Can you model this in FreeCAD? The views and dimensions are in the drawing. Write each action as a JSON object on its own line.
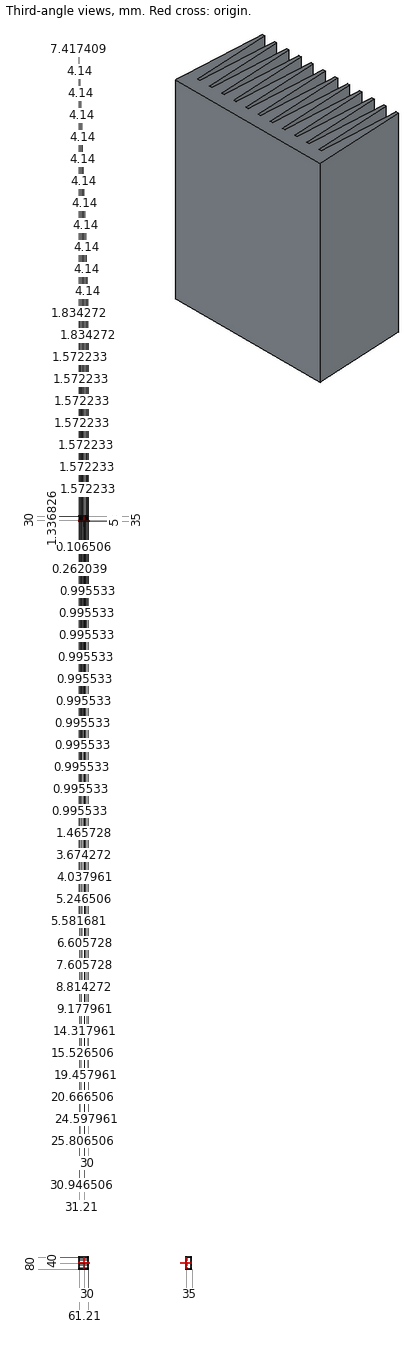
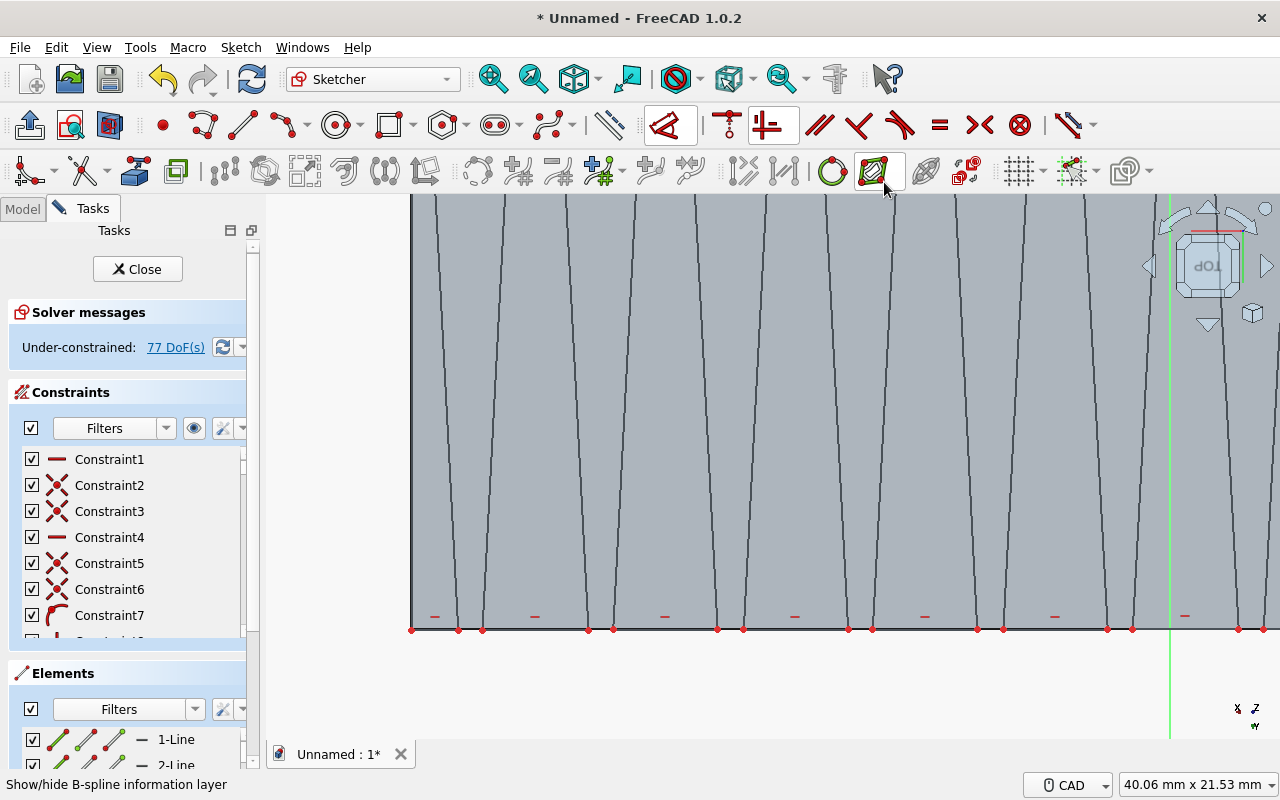
{"action": "scroll", "coordinate": [424, 630], "scroll_direction": "down", "scroll_amount": 5}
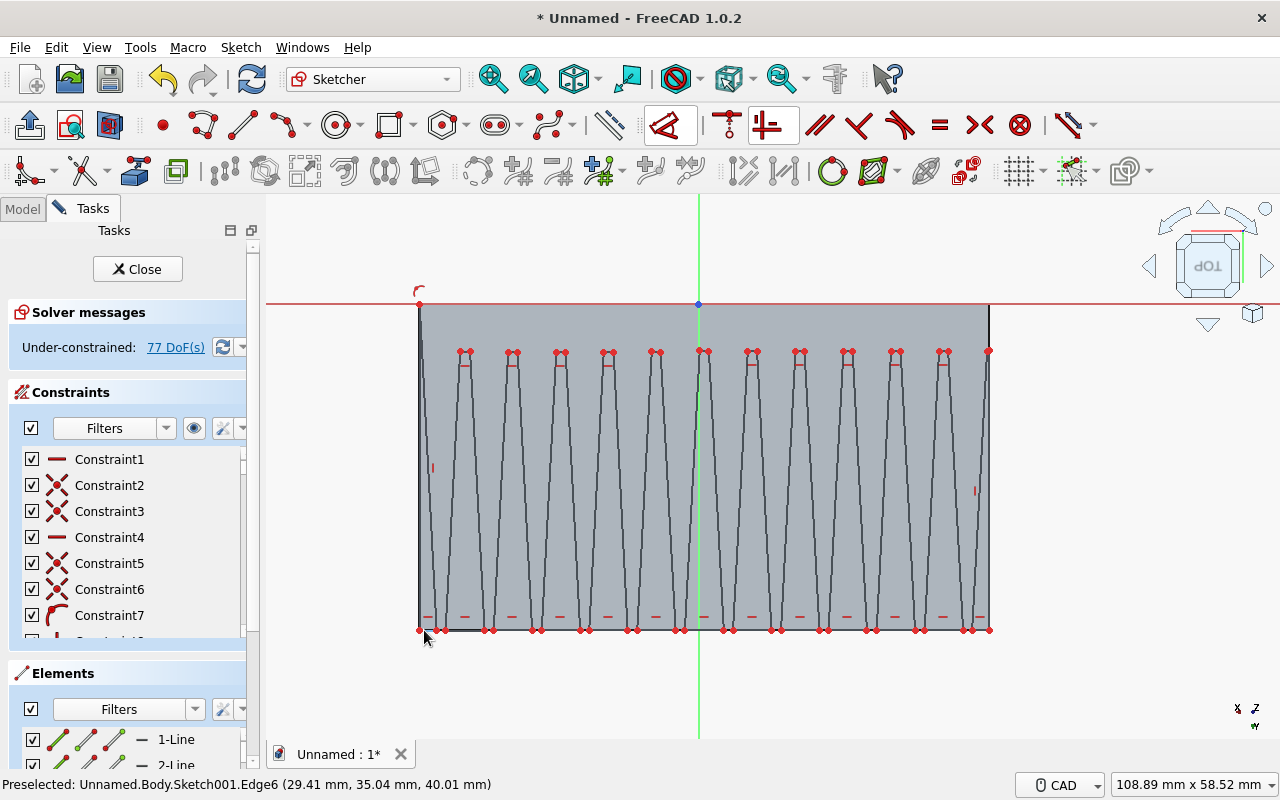
{"action": "scroll", "coordinate": [657, 352], "scroll_direction": "up", "scroll_amount": 7}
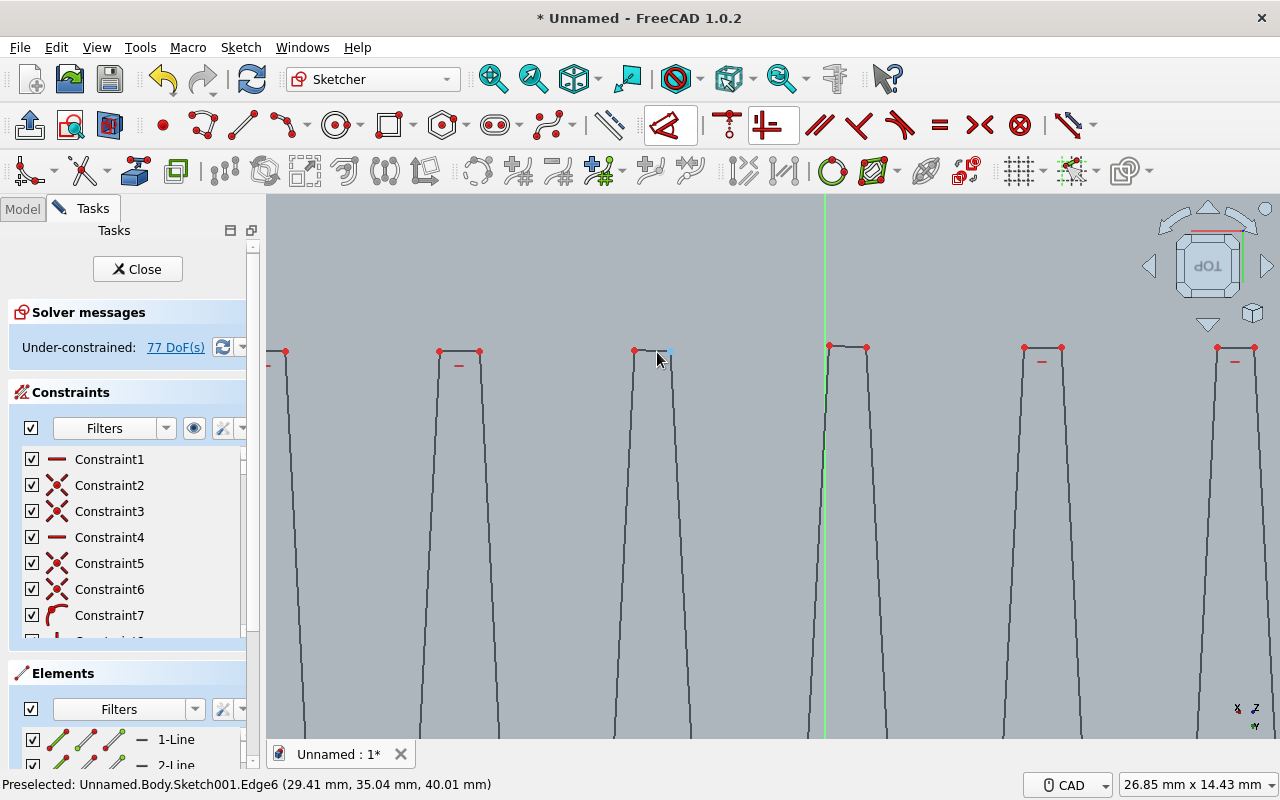
{"action": "left_click", "coordinate": [656, 351]}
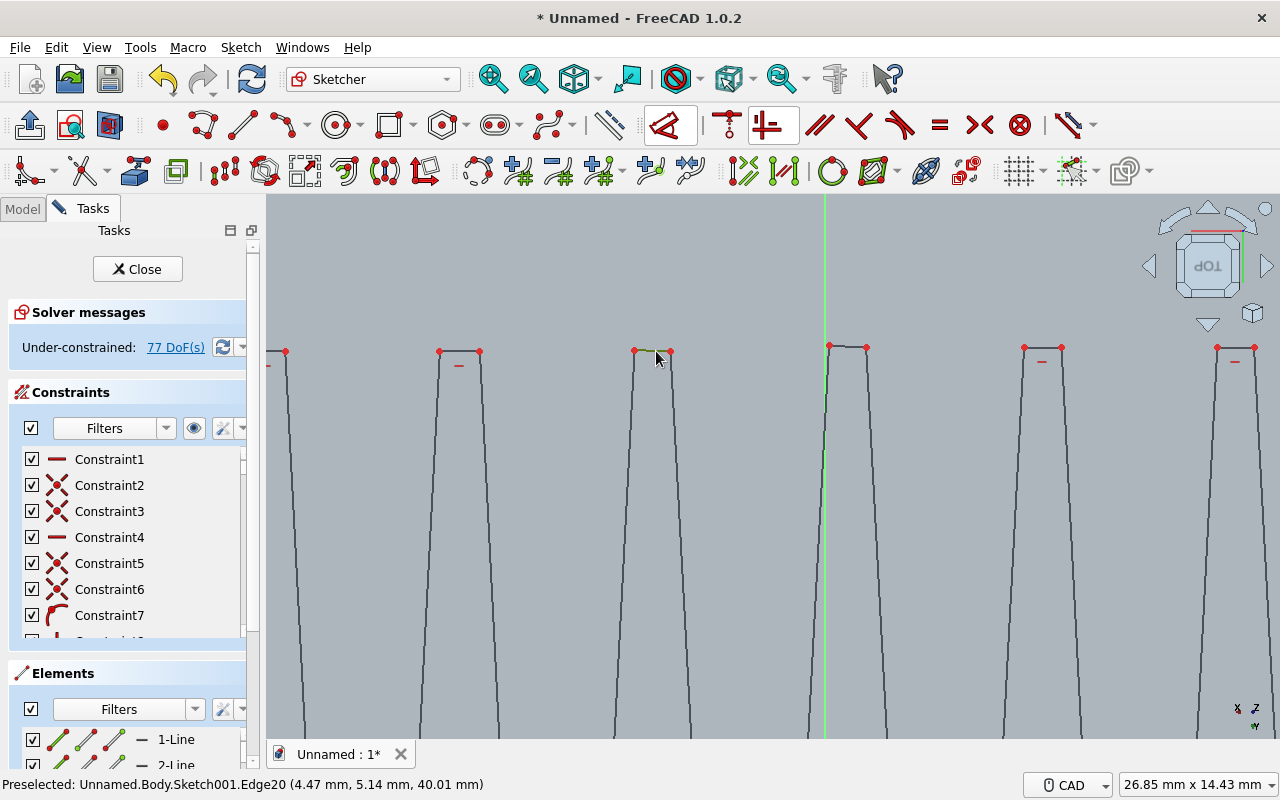
{"action": "key", "text": "h"}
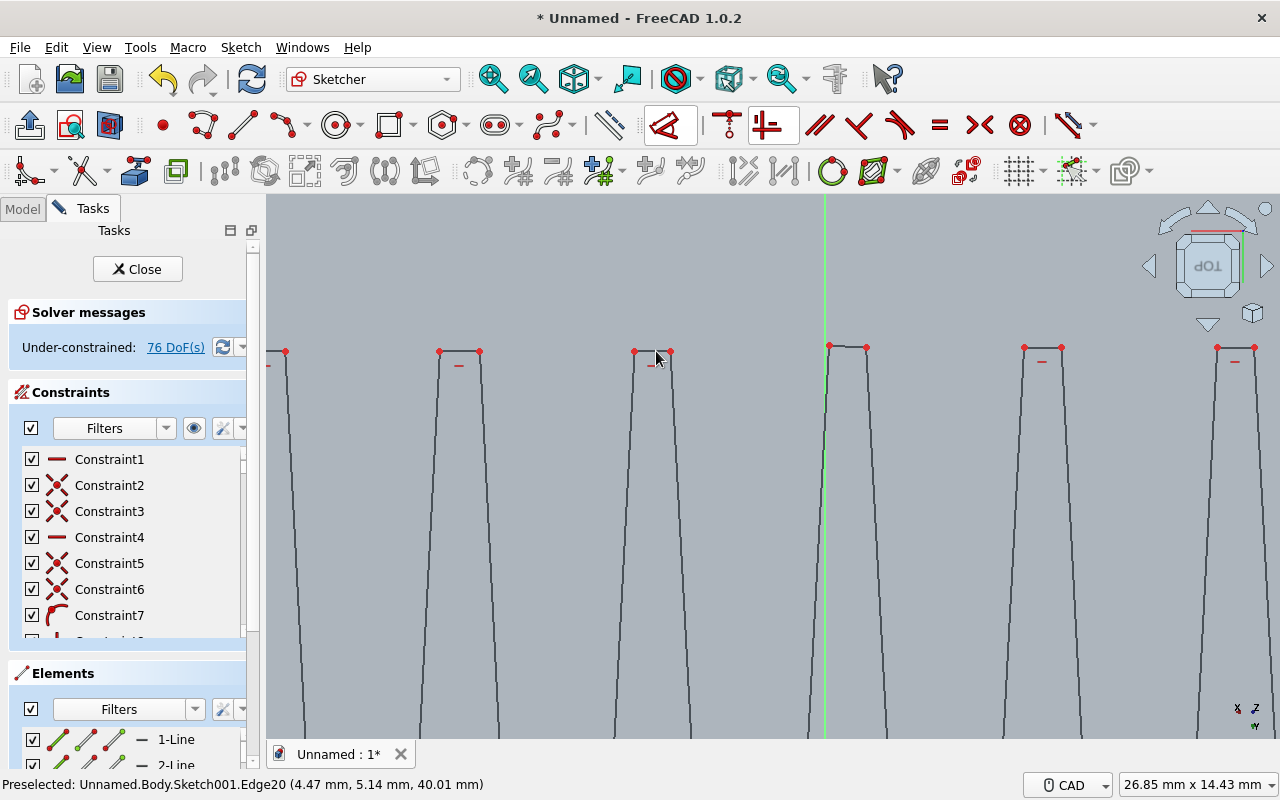
{"action": "scroll", "coordinate": [855, 347], "scroll_direction": "up", "scroll_amount": 2}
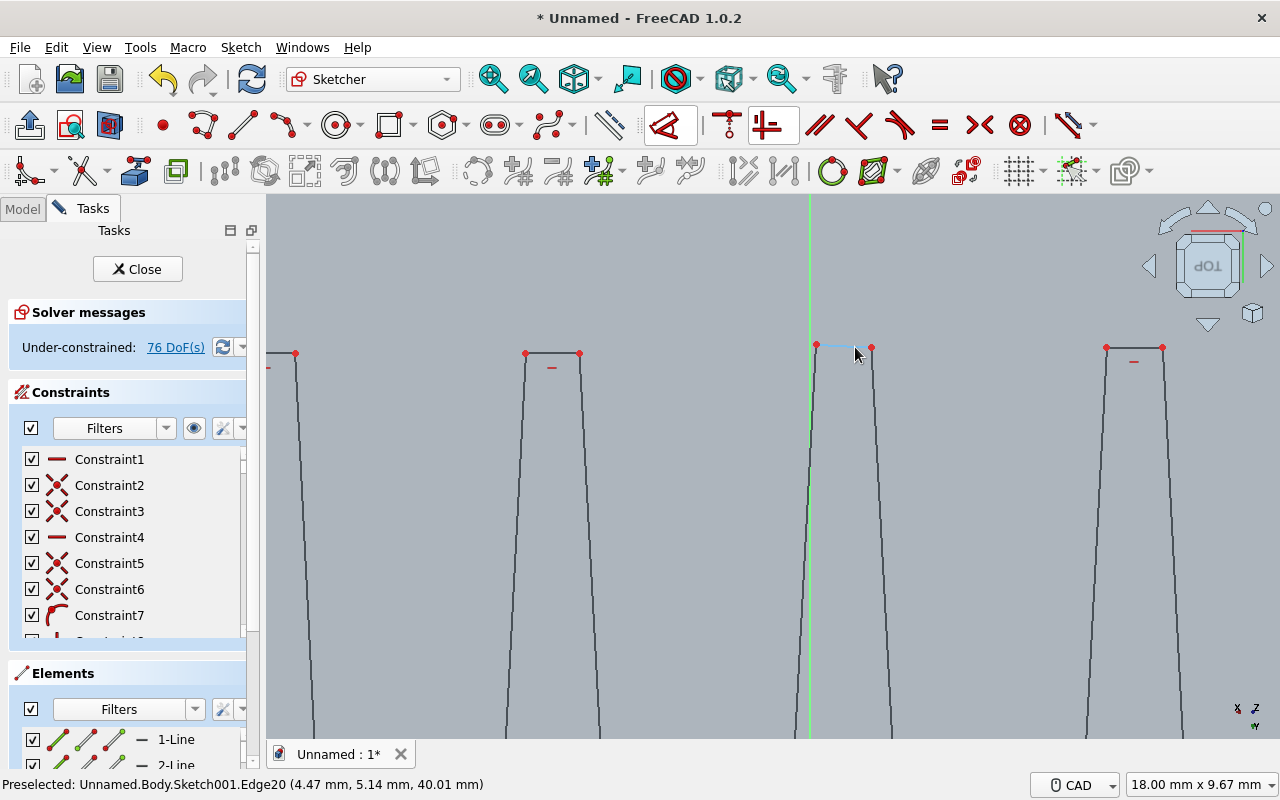
{"action": "left_click", "coordinate": [855, 347]}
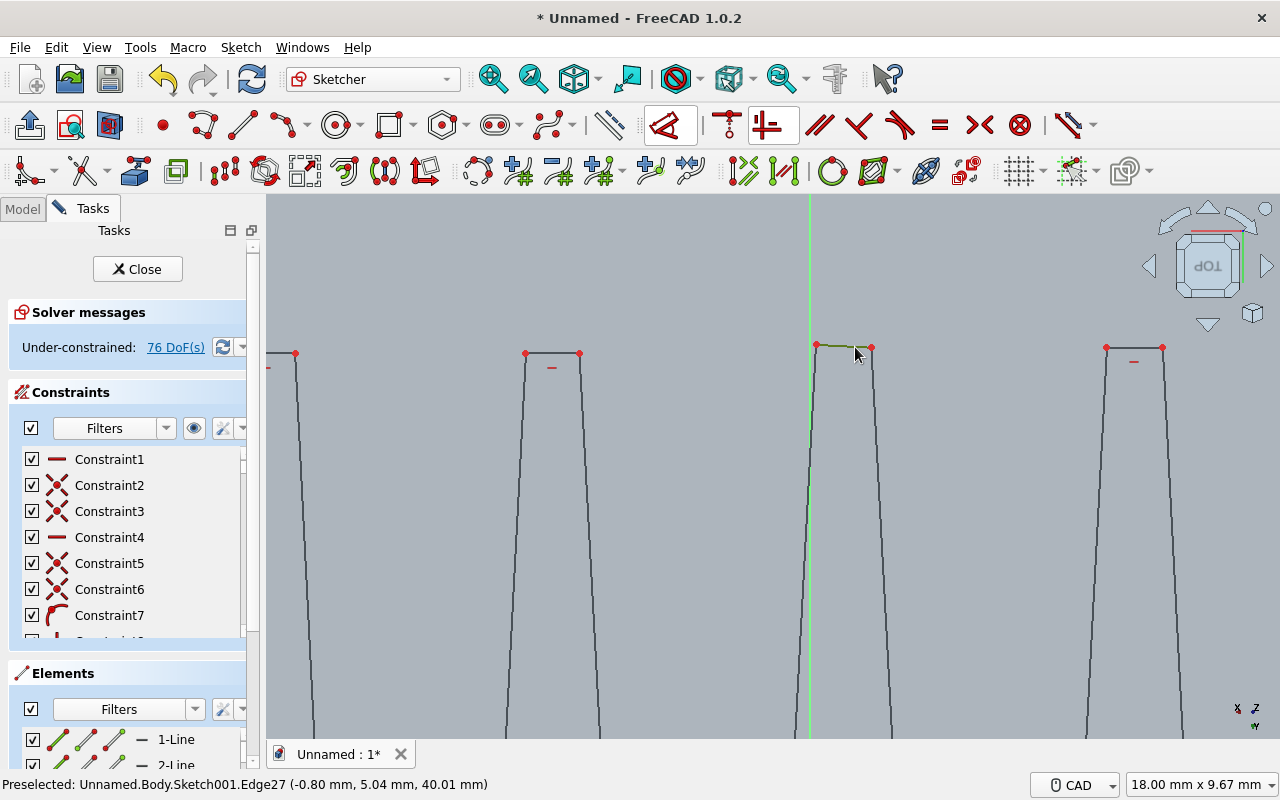
{"action": "key", "text": "h"}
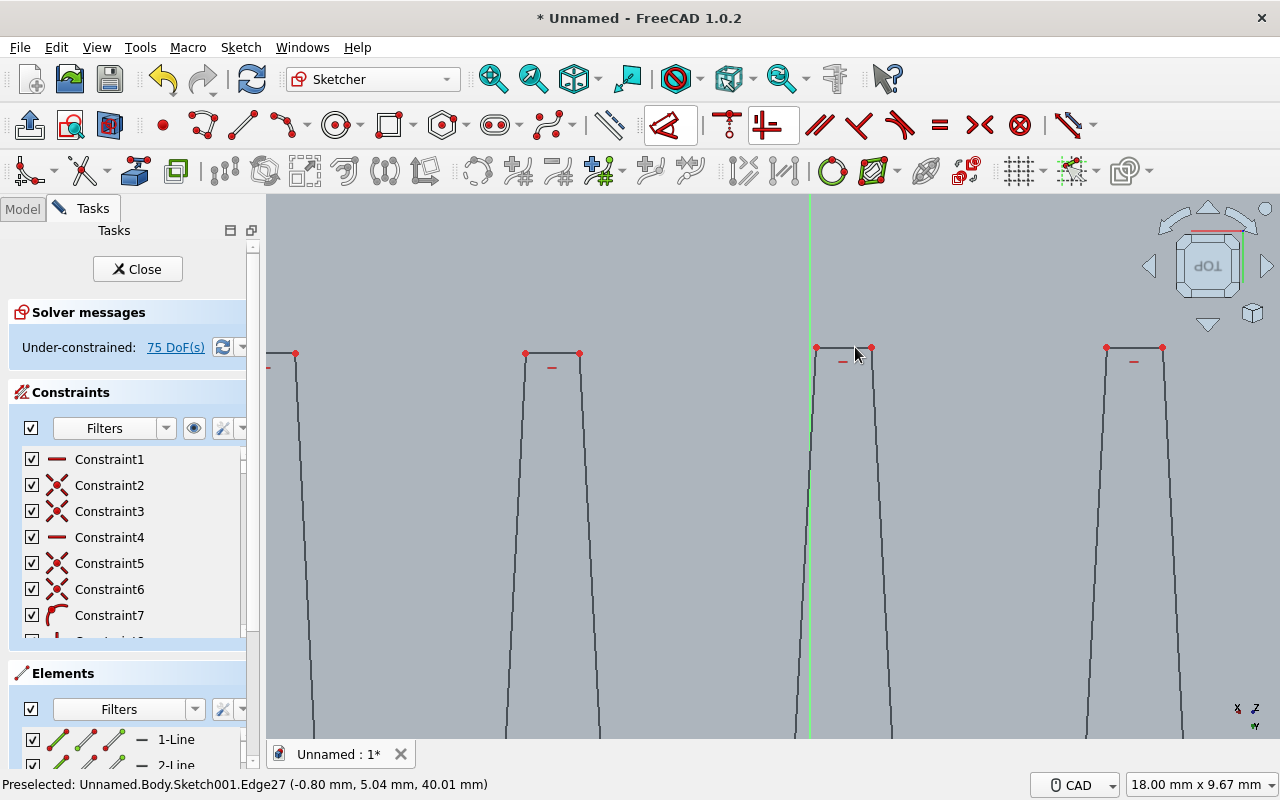
{"action": "scroll", "coordinate": [677, 351], "scroll_direction": "down", "scroll_amount": 9}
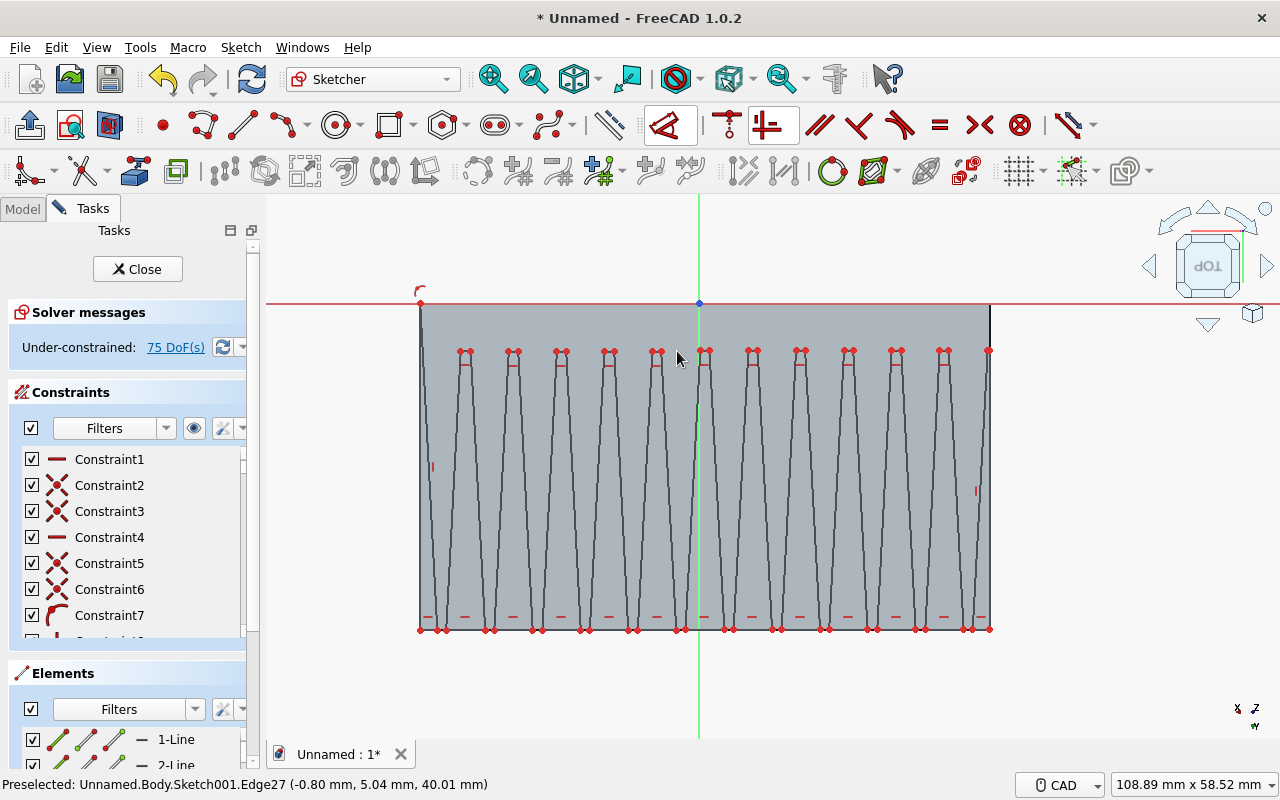
{"action": "scroll", "coordinate": [989, 350], "scroll_direction": "up", "scroll_amount": 13}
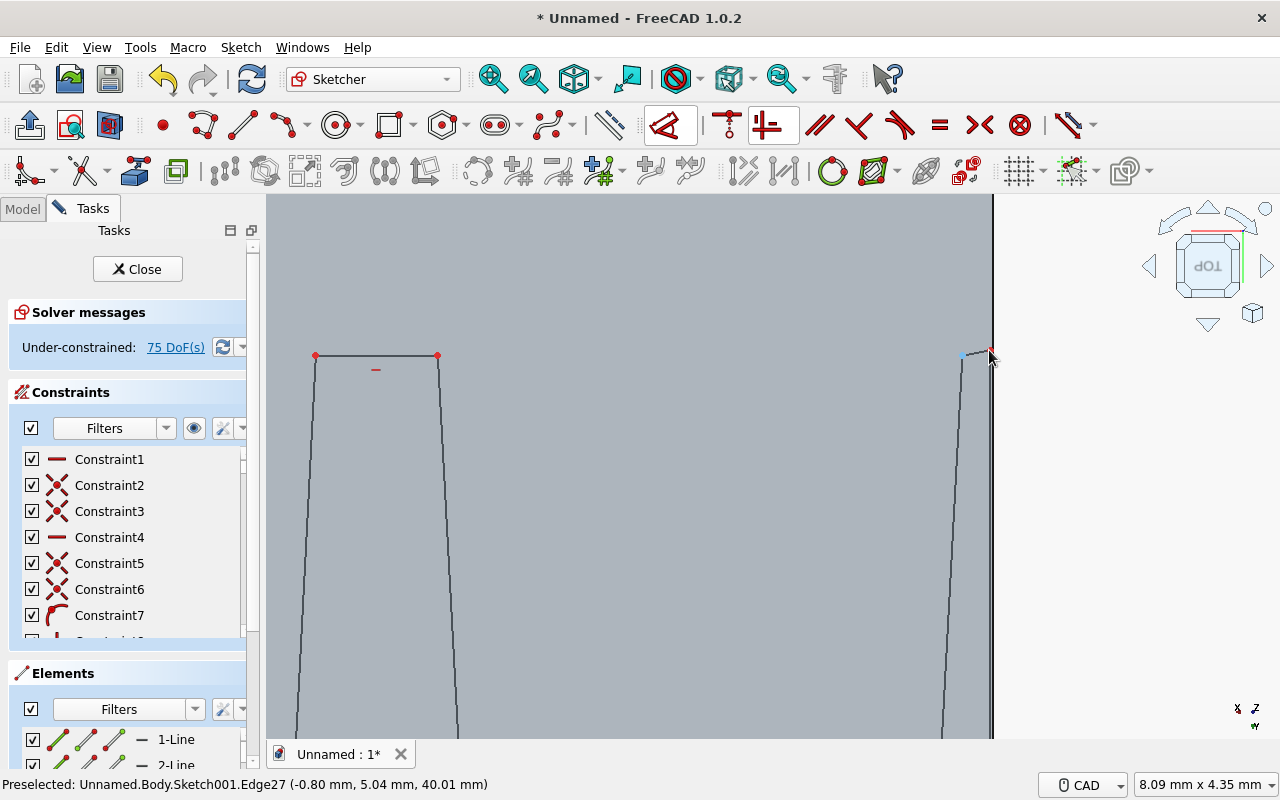
{"action": "left_click", "coordinate": [976, 353]}